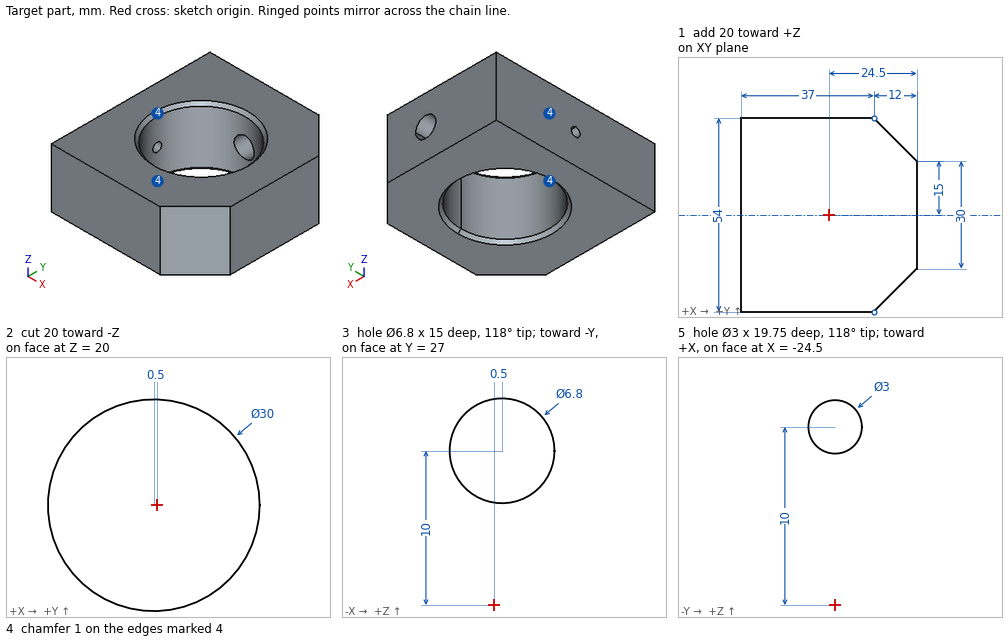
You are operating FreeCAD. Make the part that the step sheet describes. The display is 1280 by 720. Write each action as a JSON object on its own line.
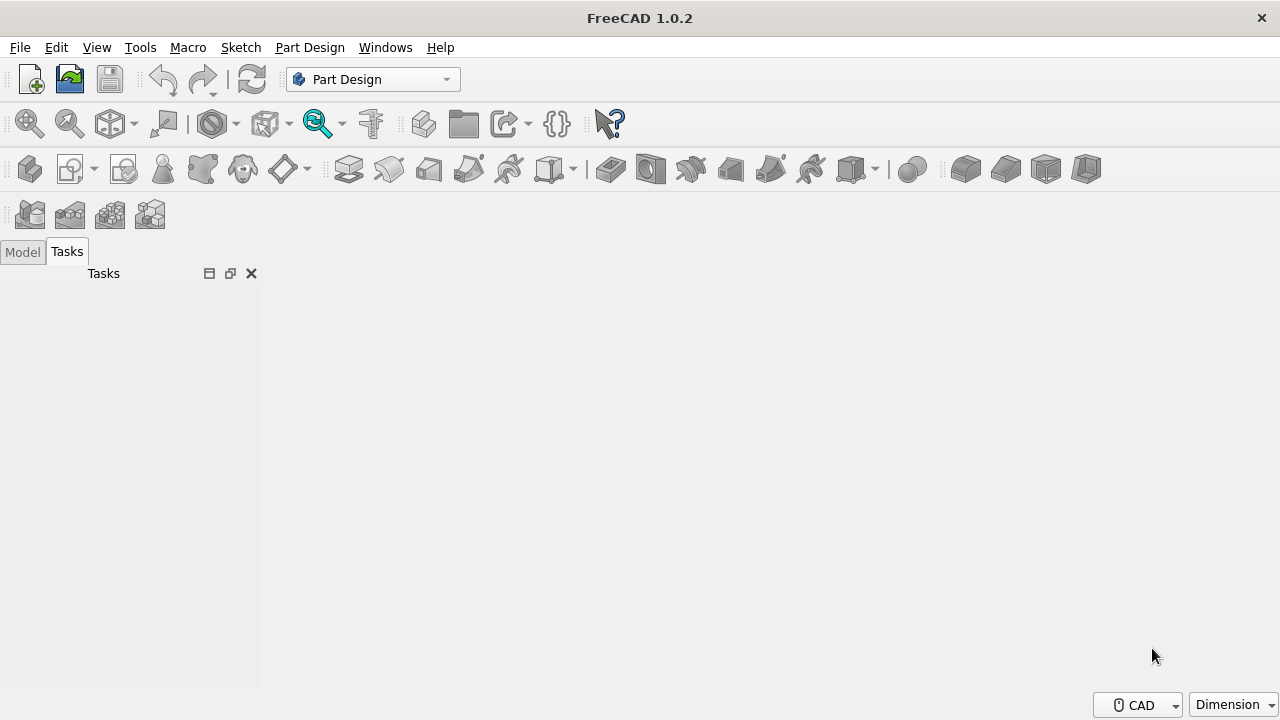
{"action": "left_click", "coordinate": [30, 80]}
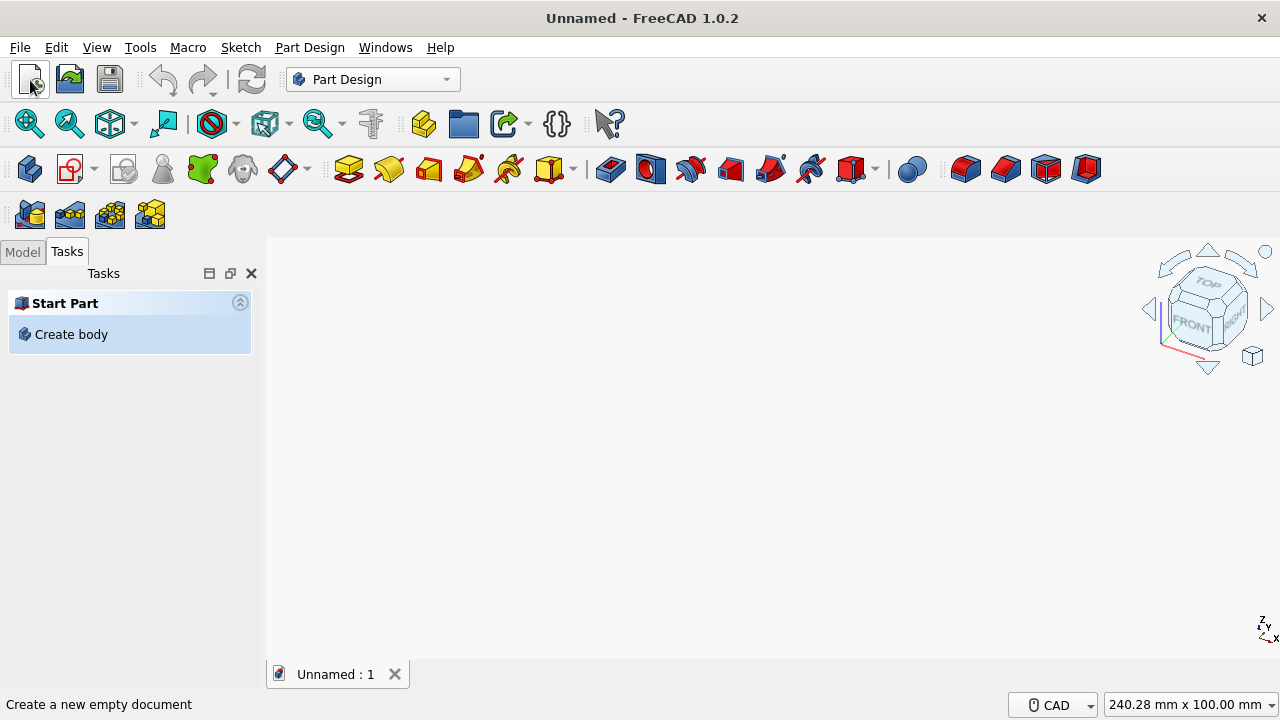
{"action": "left_click", "coordinate": [70, 170]}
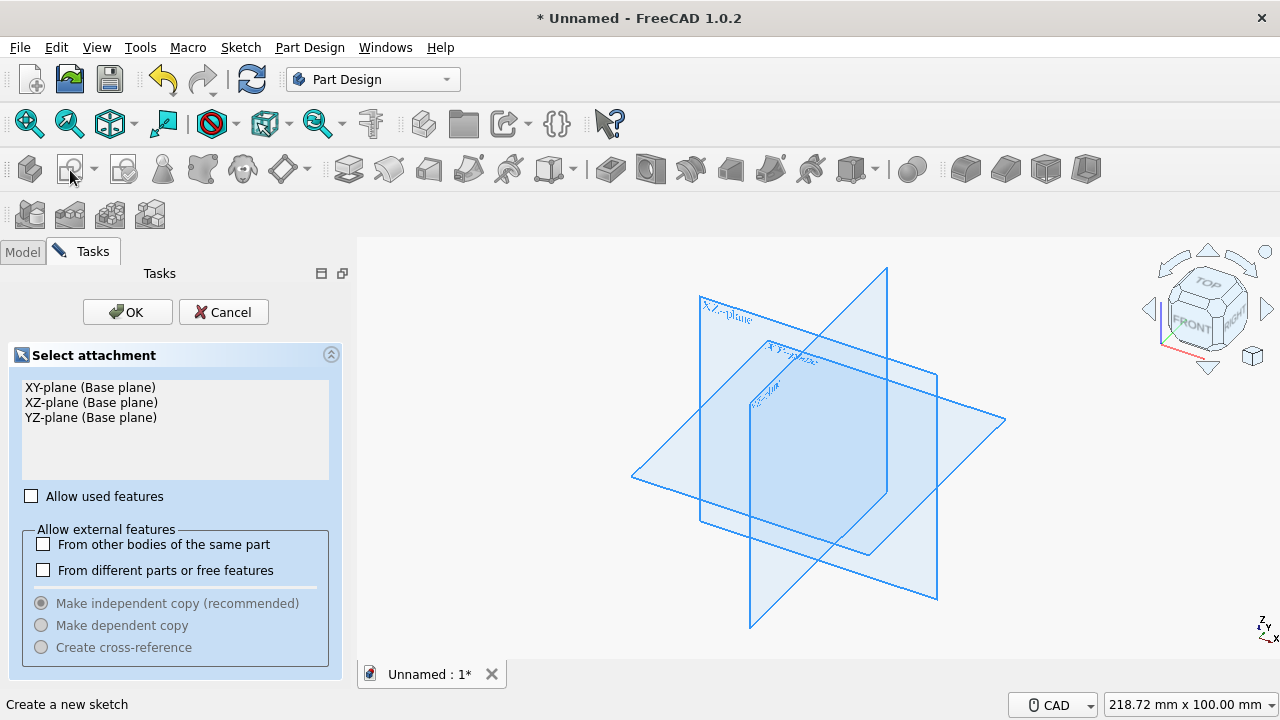
{"action": "left_click", "coordinate": [82, 388]}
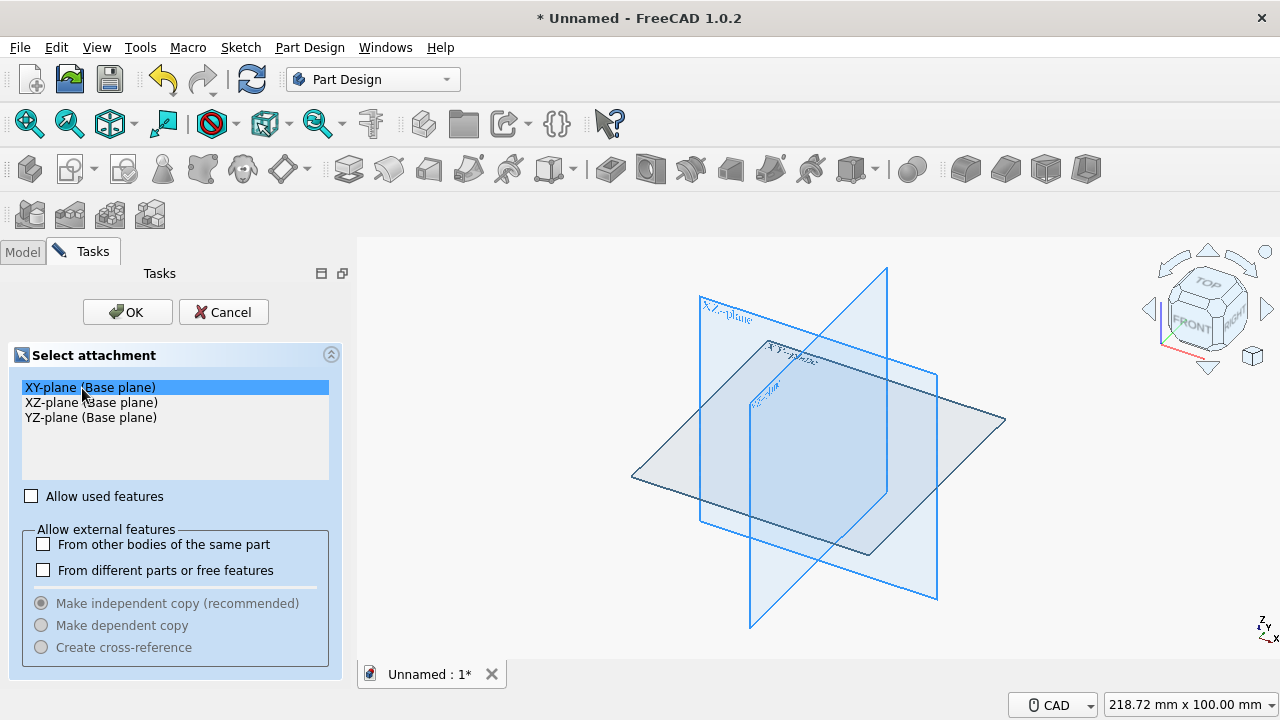
{"action": "left_click", "coordinate": [128, 312]}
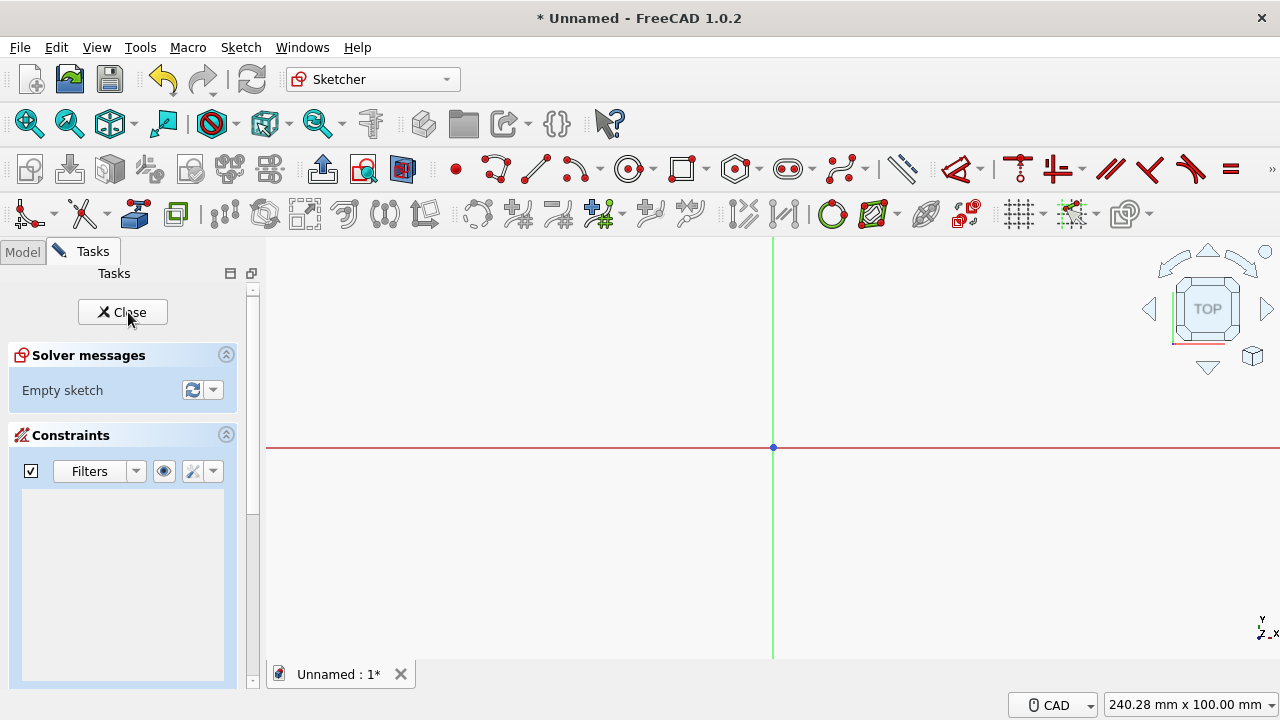
{"action": "left_click", "coordinate": [496, 170]}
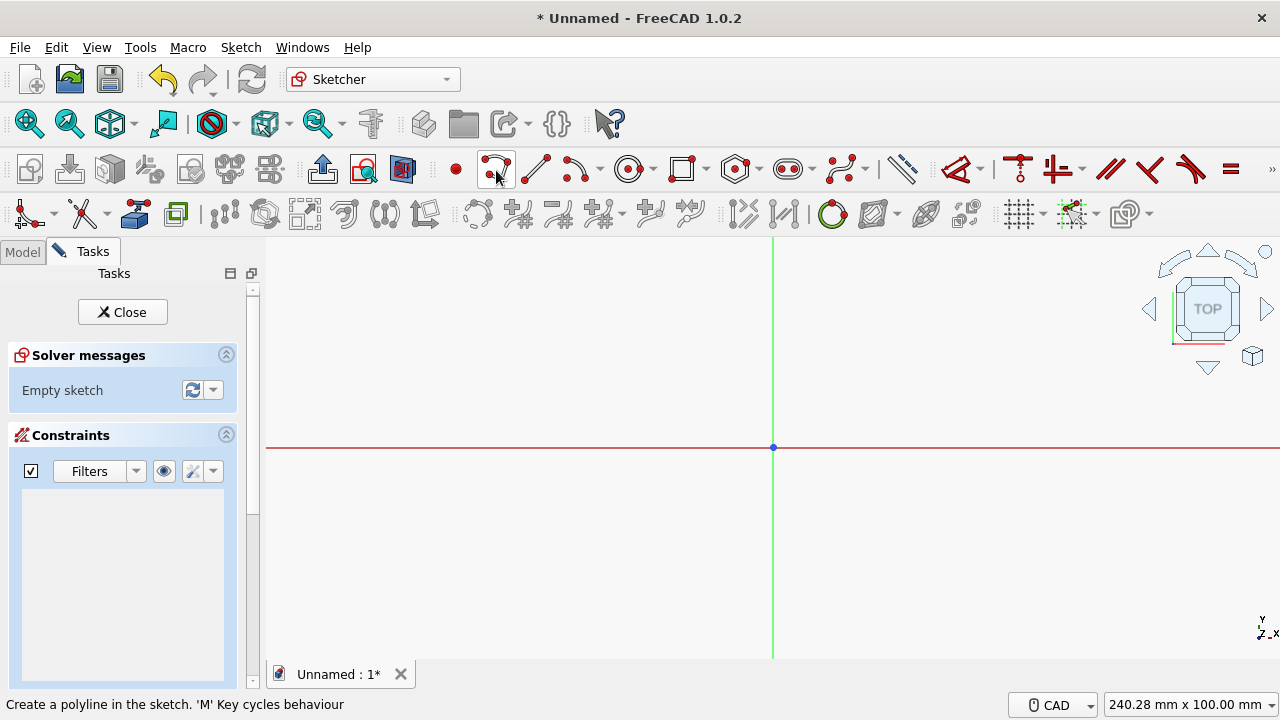
{"action": "left_click", "coordinate": [876, 385]}
{"action": "left_click", "coordinate": [826, 334]}
{"action": "left_click", "coordinate": [670, 334]}
{"action": "left_click", "coordinate": [670, 562]}
{"action": "left_click", "coordinate": [826, 562]}
{"action": "left_click", "coordinate": [876, 511]}
{"action": "left_click", "coordinate": [876, 386]}
{"action": "key", "text": "Escape"}
{"action": "key", "text": "Escape"}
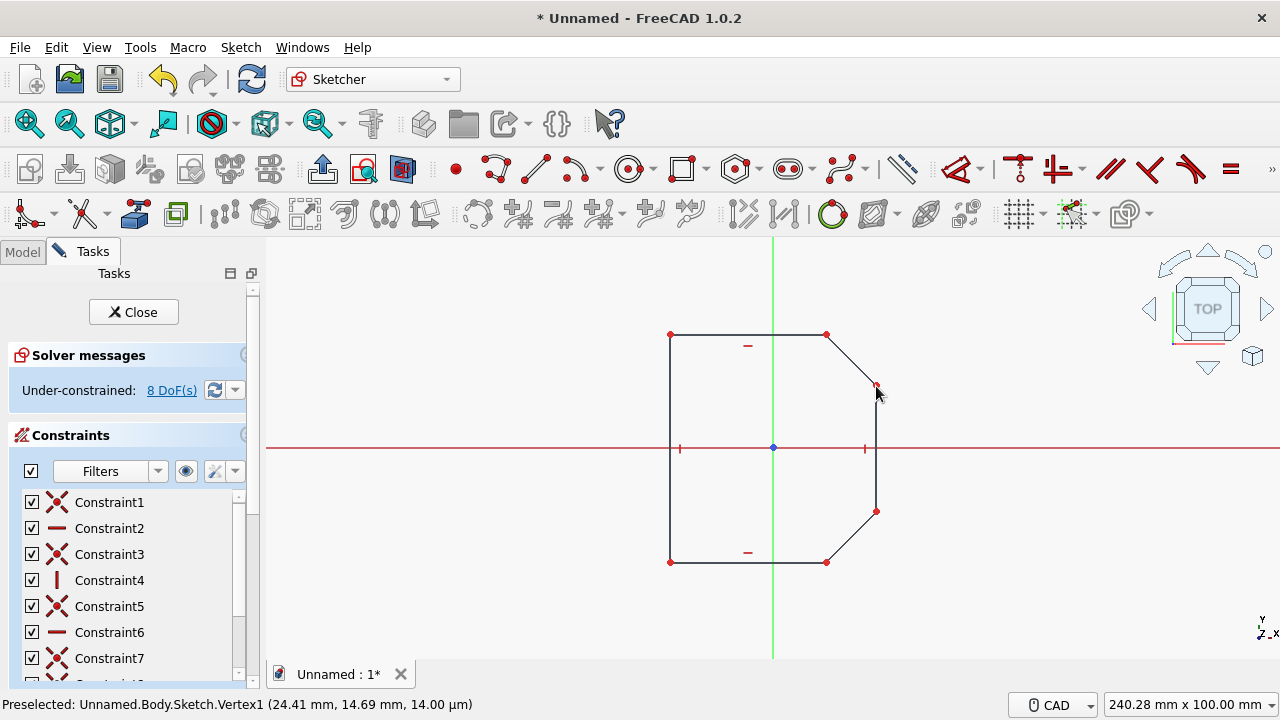
{"action": "left_click", "coordinate": [826, 335]}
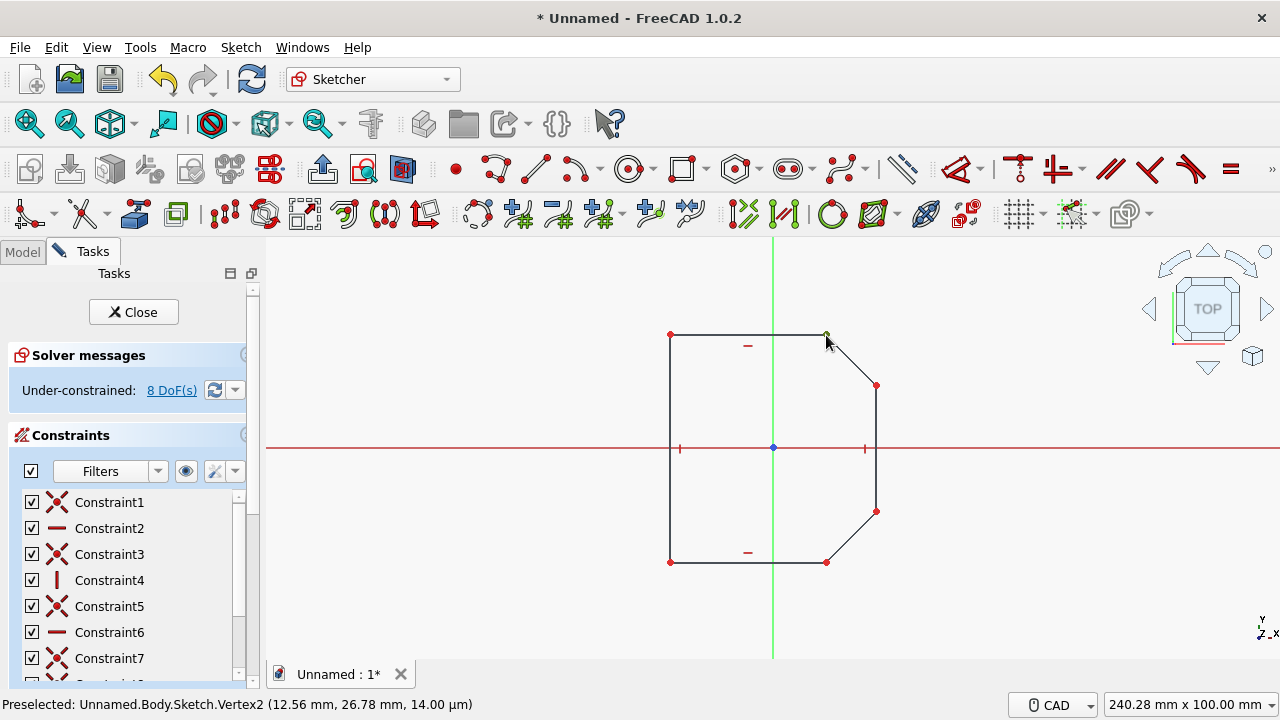
{"action": "left_click", "coordinate": [826, 563]}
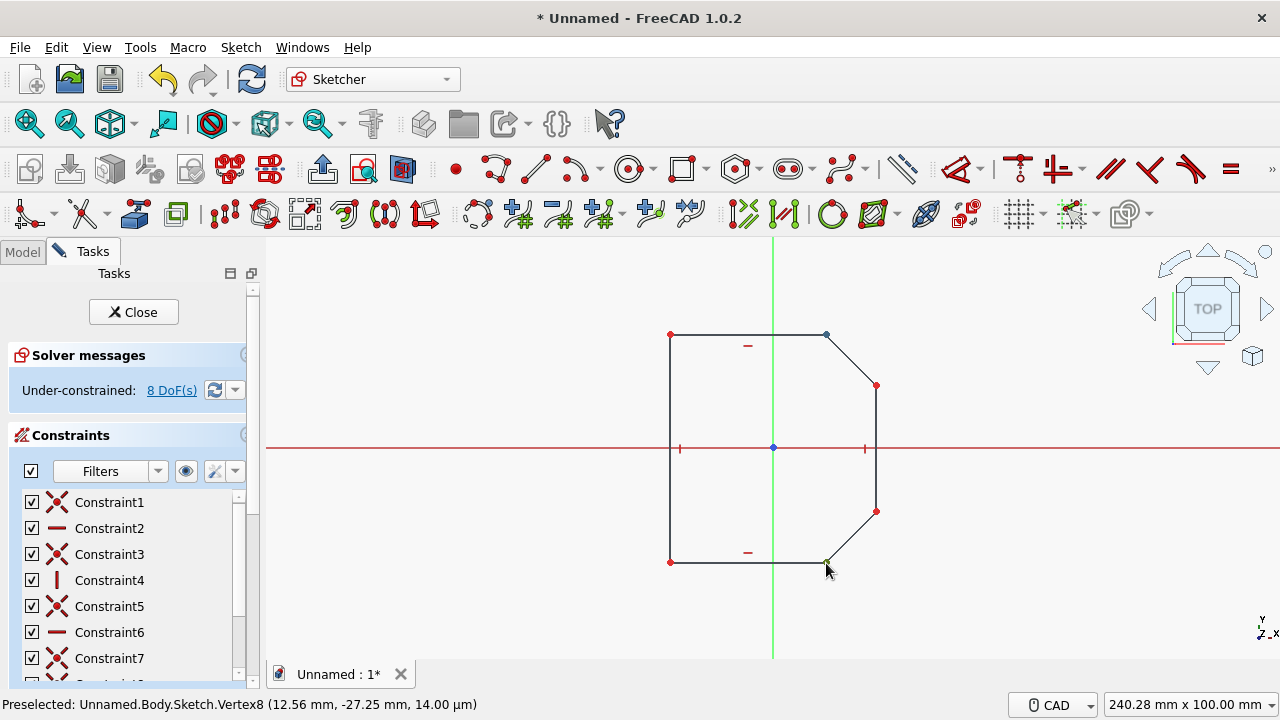
{"action": "left_click", "coordinate": [353, 448]}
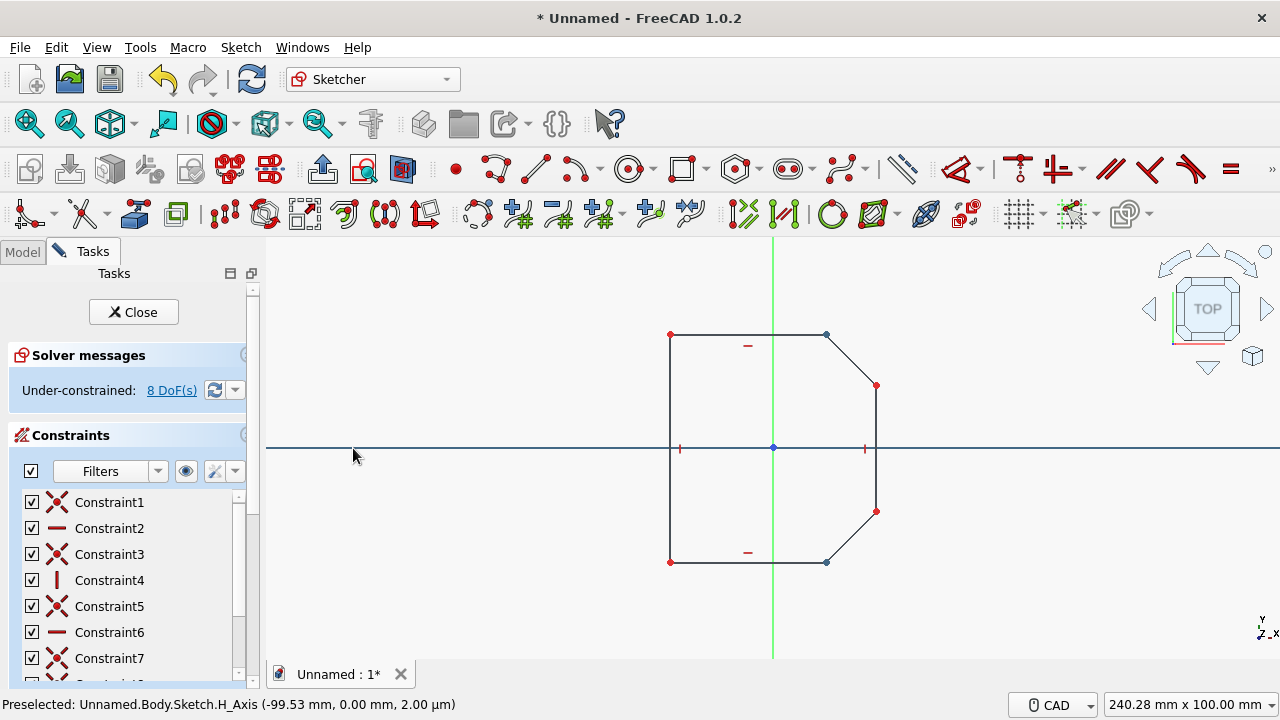
{"action": "key", "text": "s"}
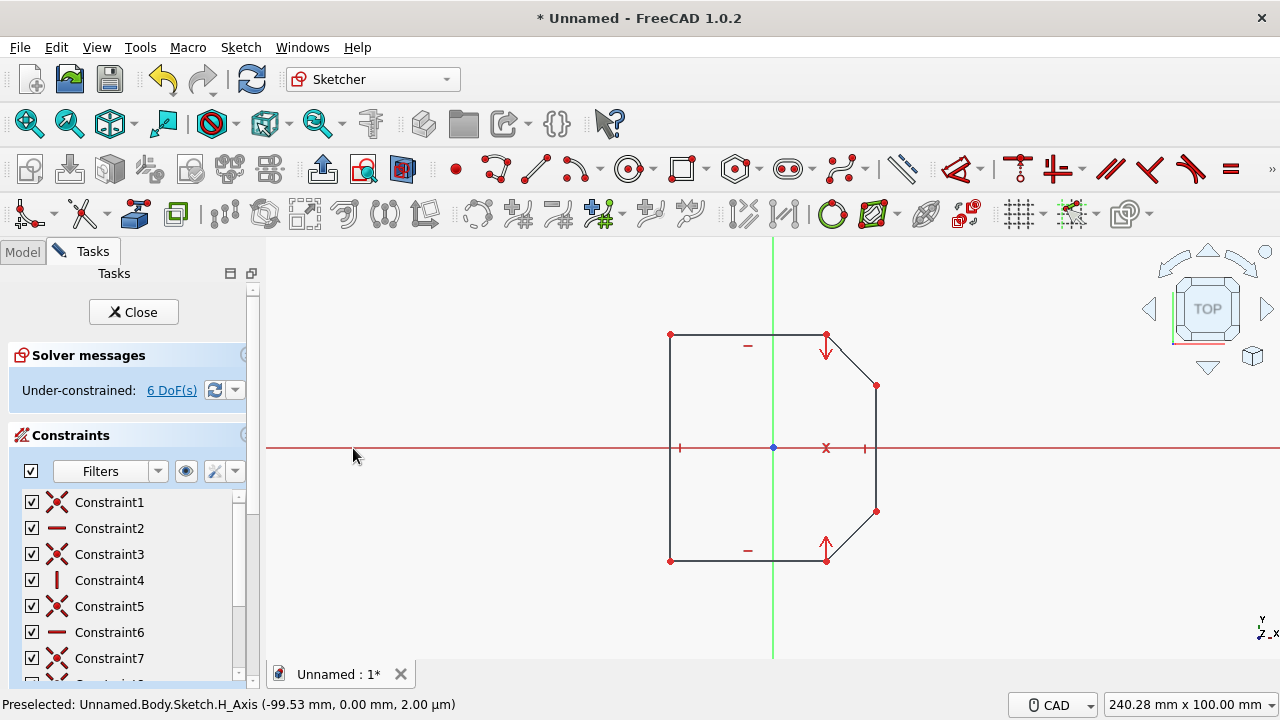
{"action": "key", "text": "d"}